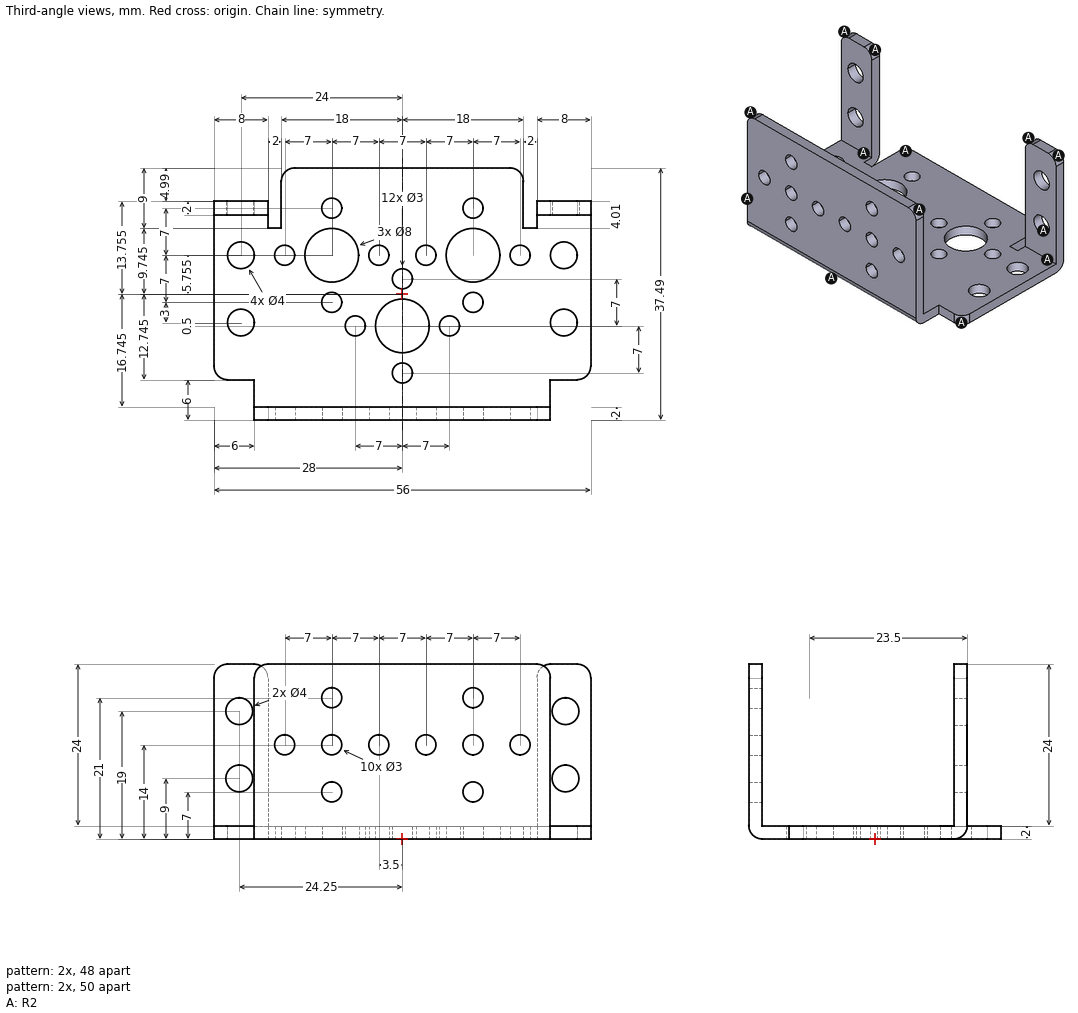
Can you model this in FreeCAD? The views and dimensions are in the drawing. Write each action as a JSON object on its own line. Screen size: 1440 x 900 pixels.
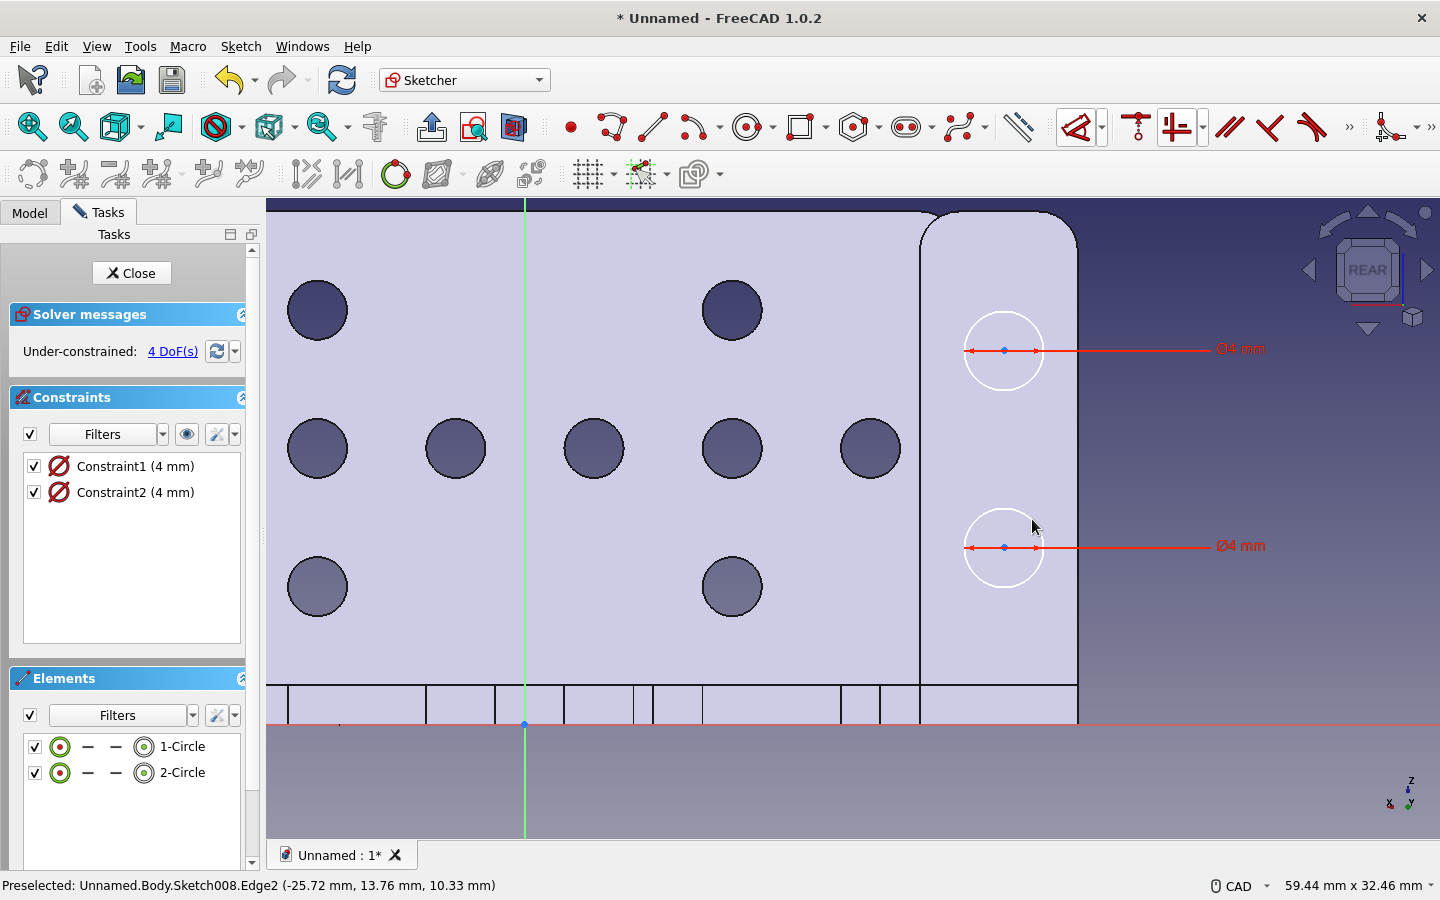
{"action": "left_click", "coordinate": [1004, 351]}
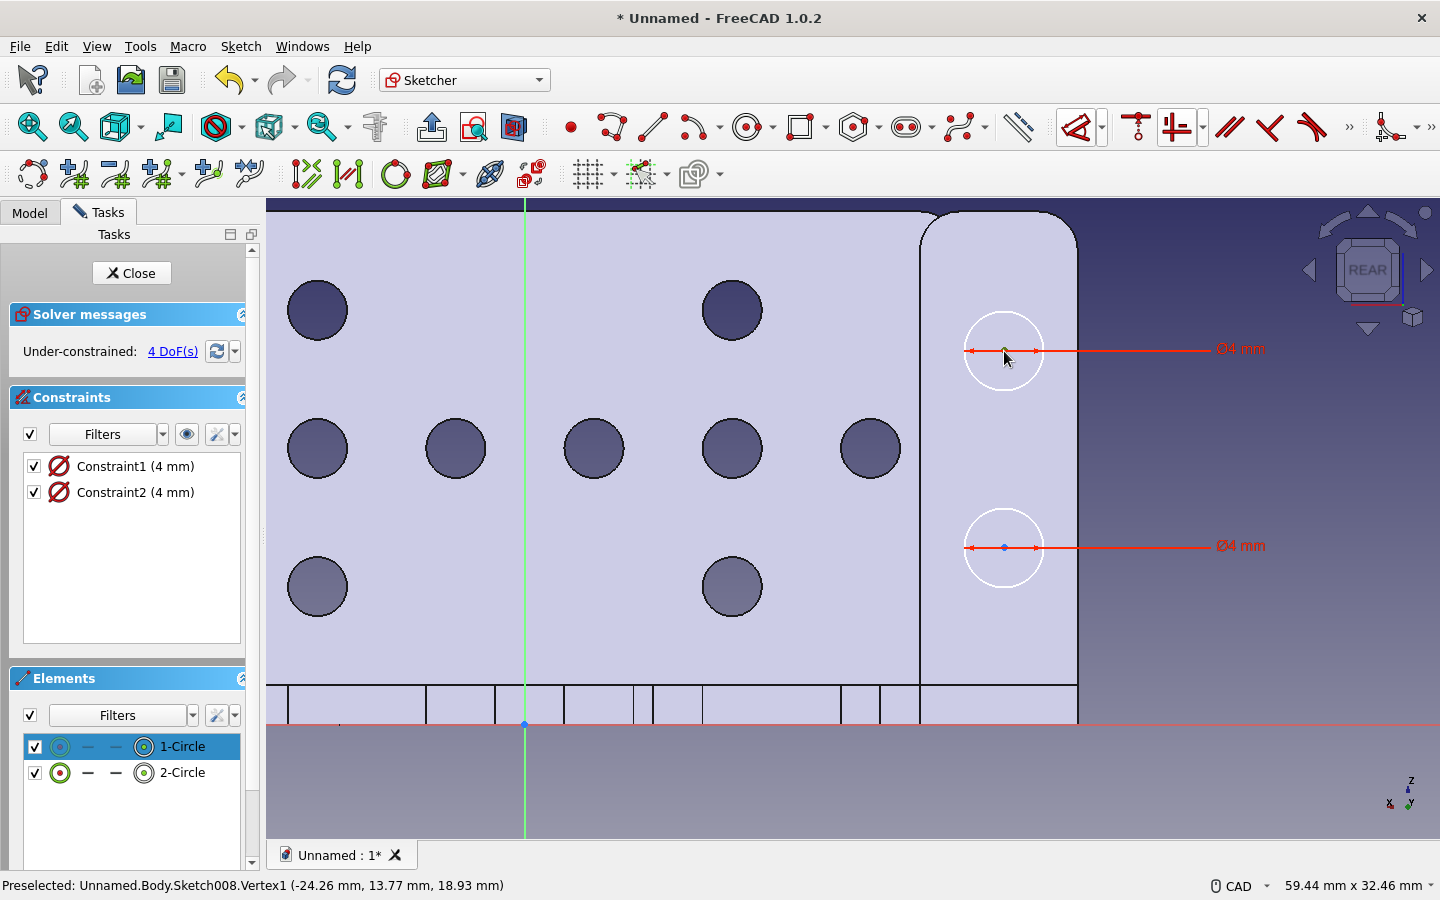
{"action": "left_click", "coordinate": [1004, 548]}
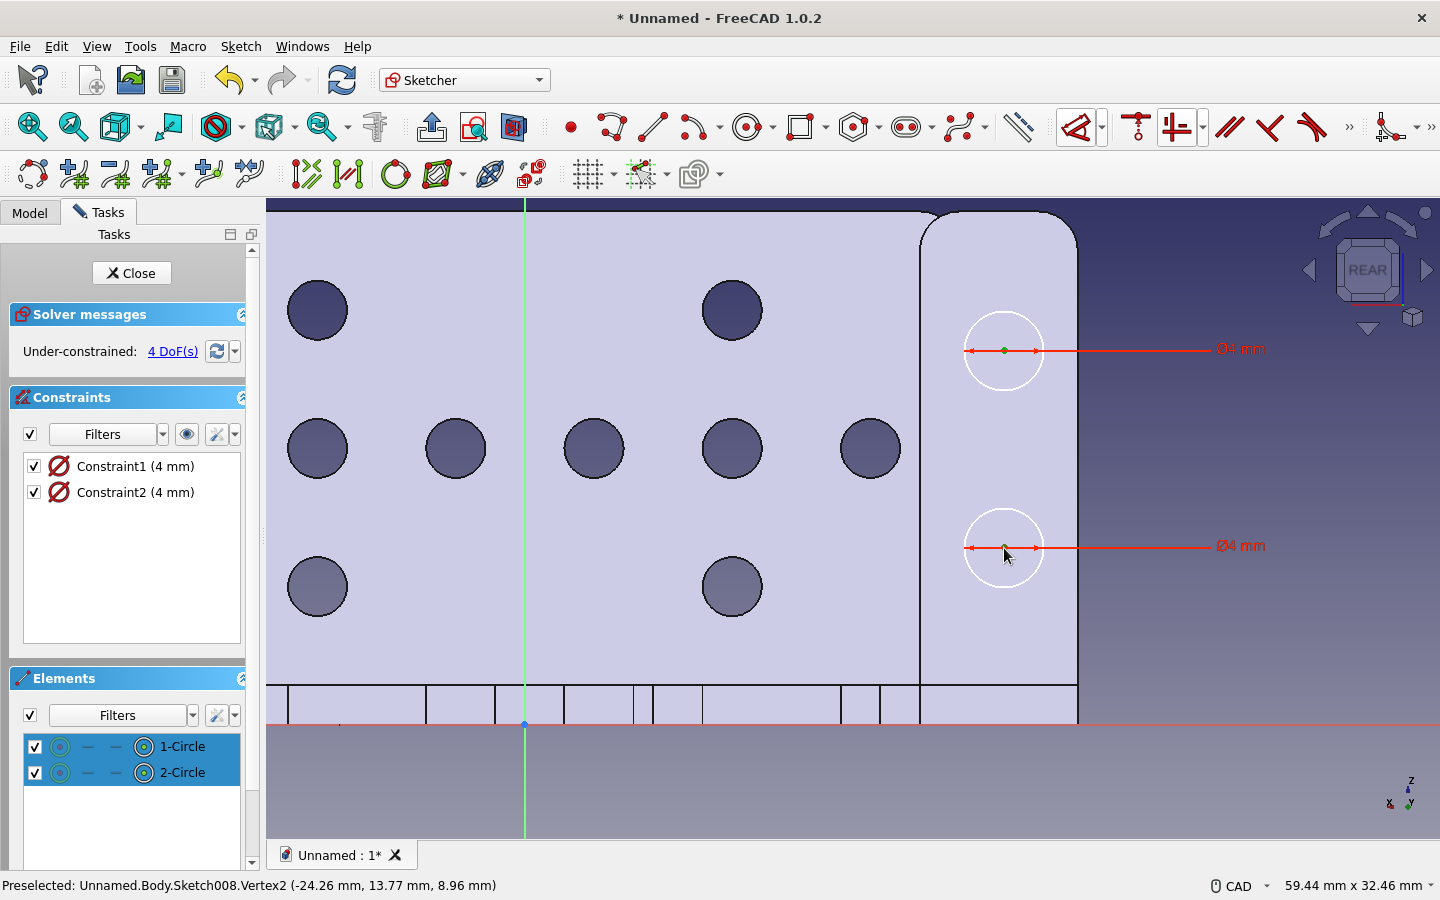
{"action": "key", "text": "v"}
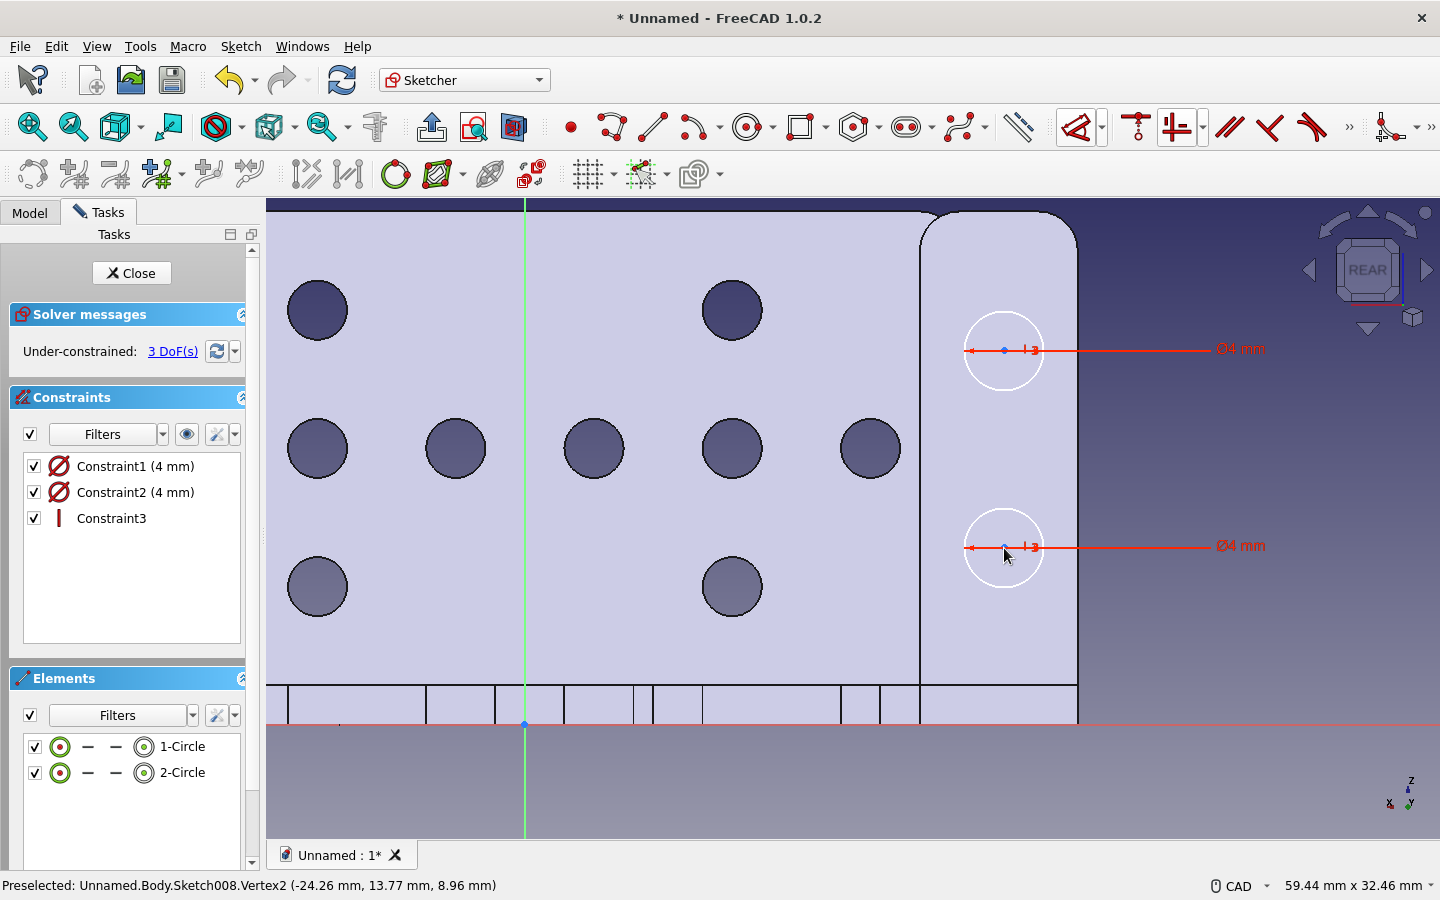
{"action": "left_click", "coordinate": [1004, 548]}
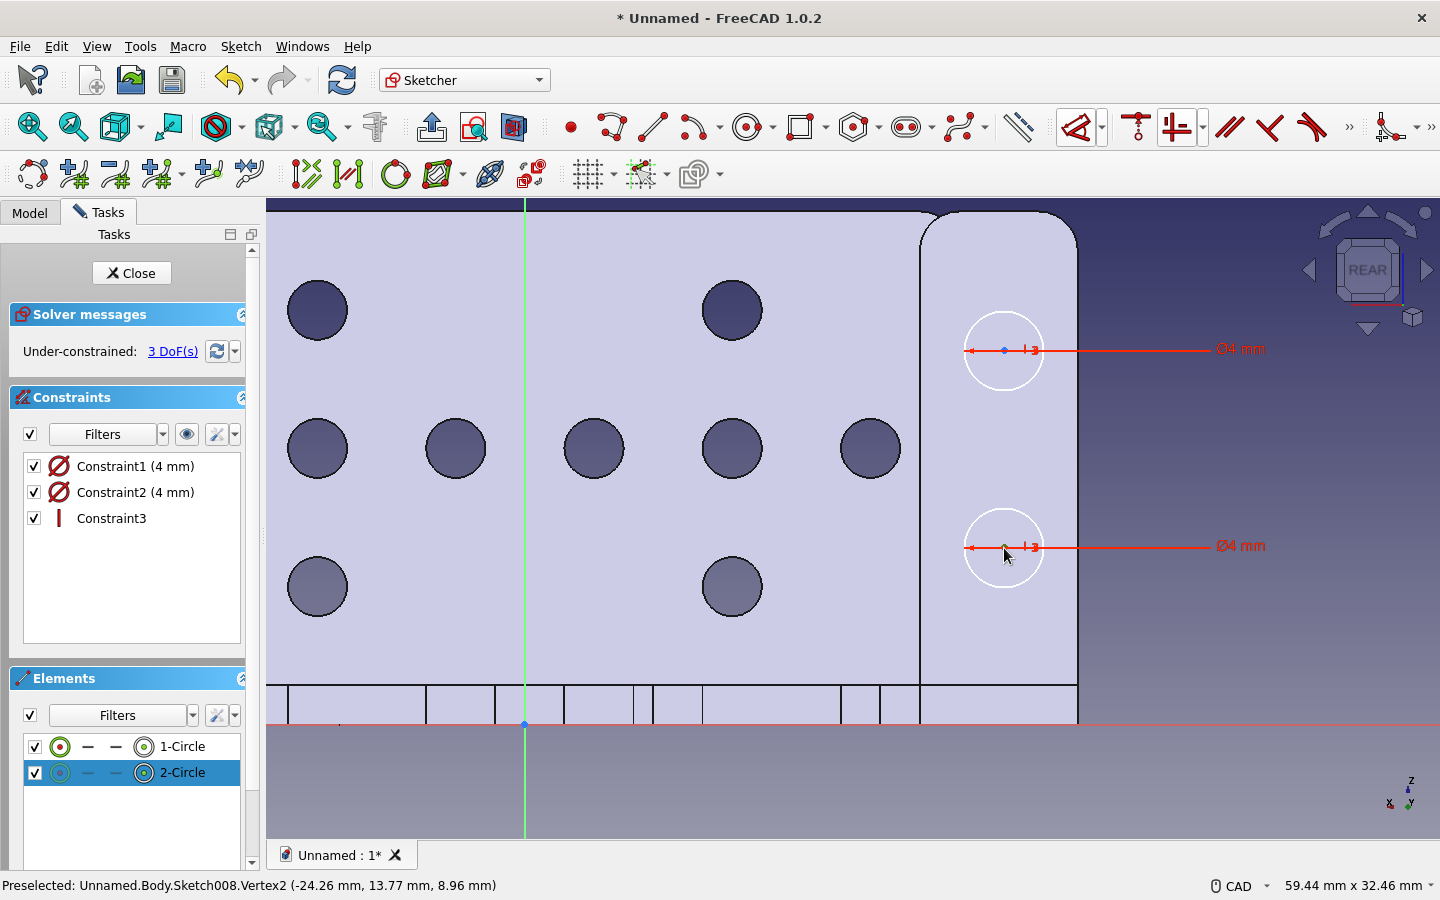
{"action": "left_click", "coordinate": [1102, 128]}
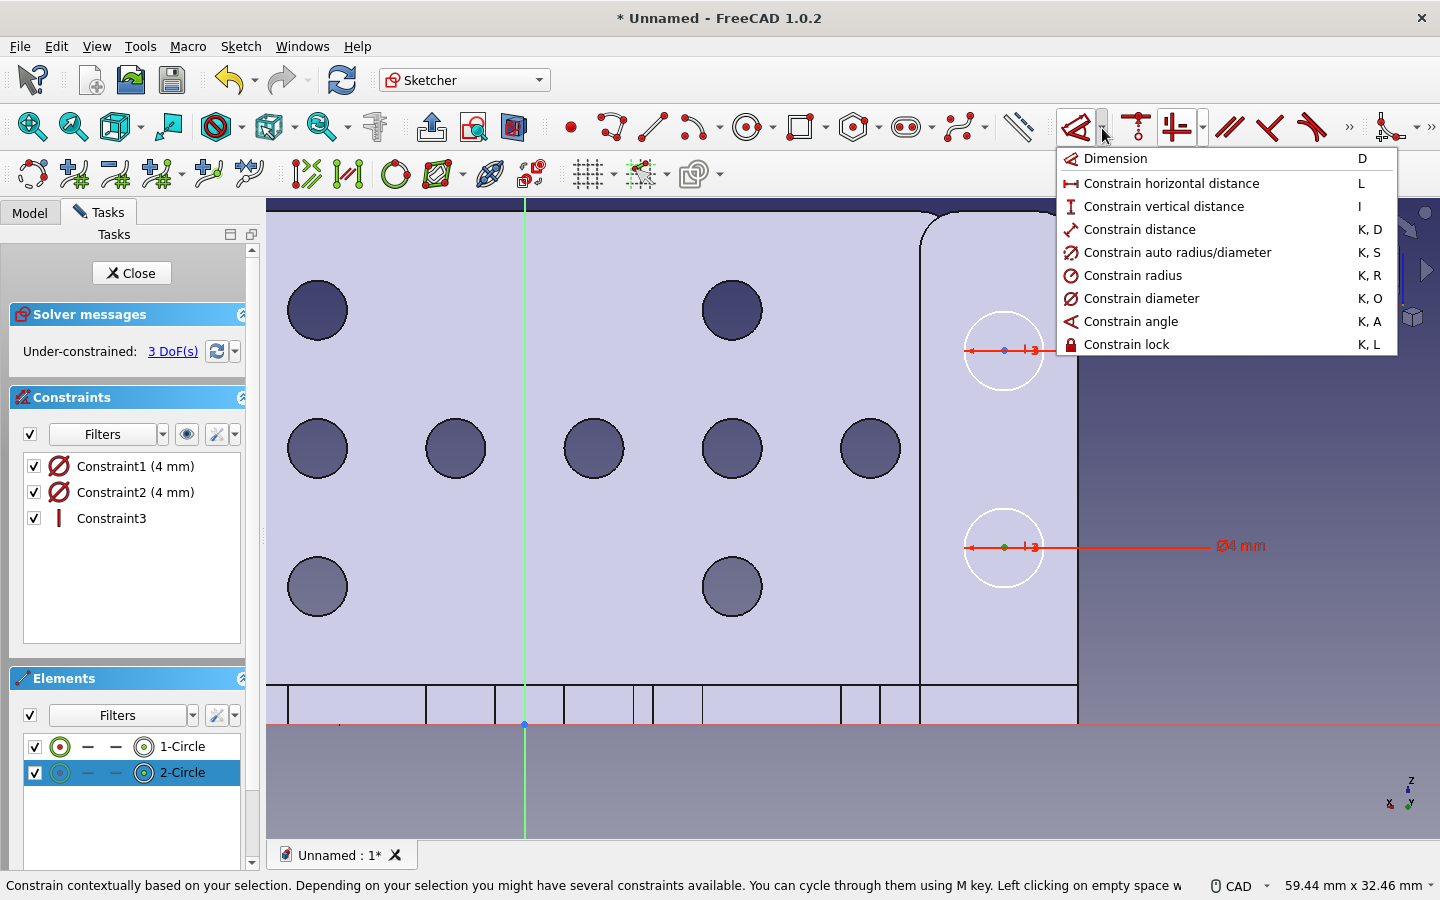
{"action": "left_click", "coordinate": [1227, 206]}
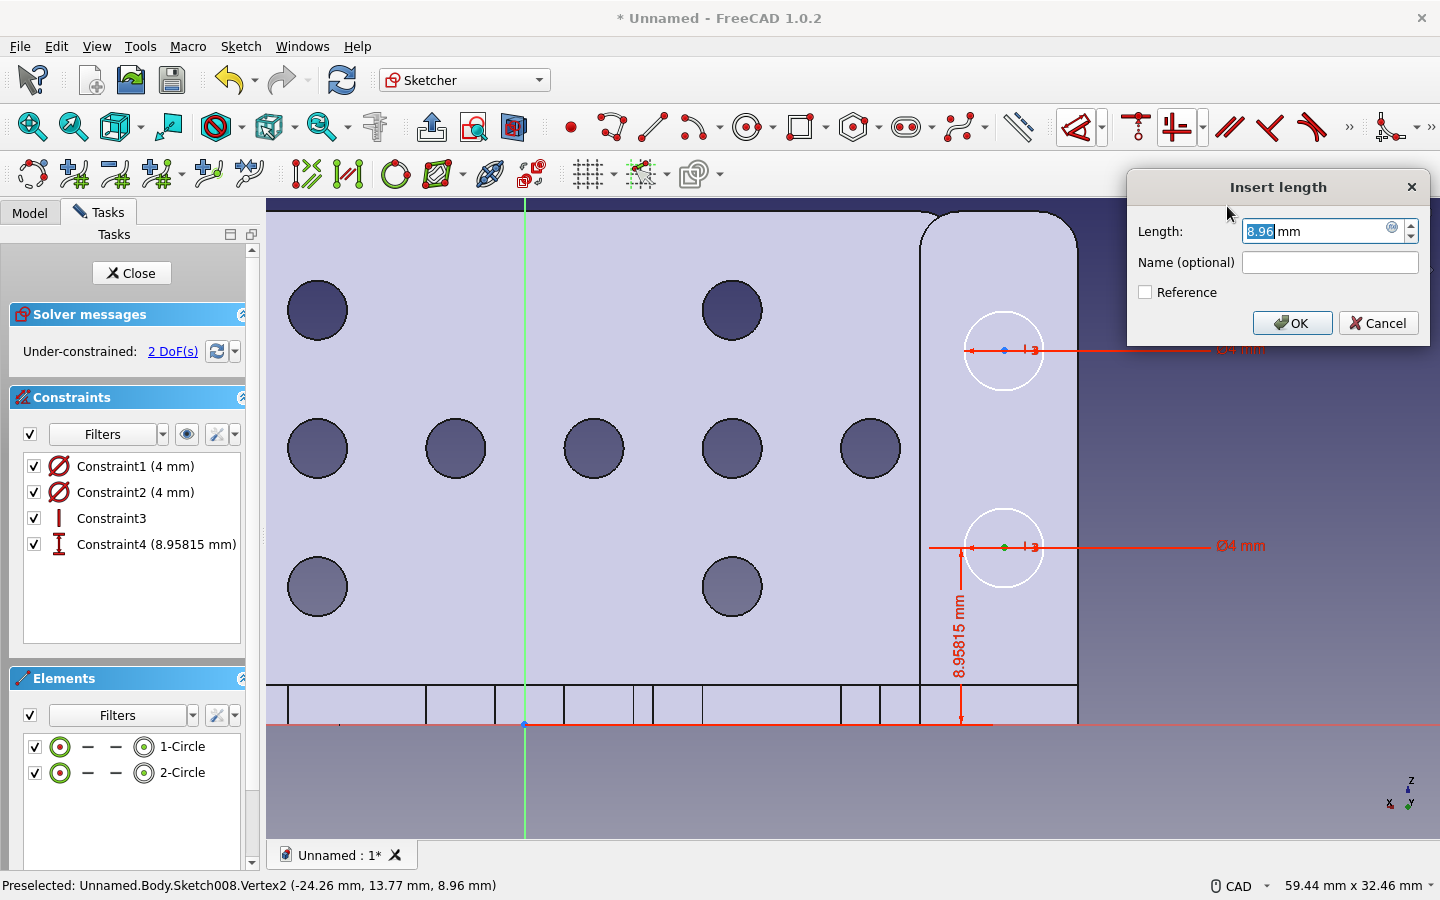
{"action": "type", "text": "9"}
{"action": "key", "text": "Return"}